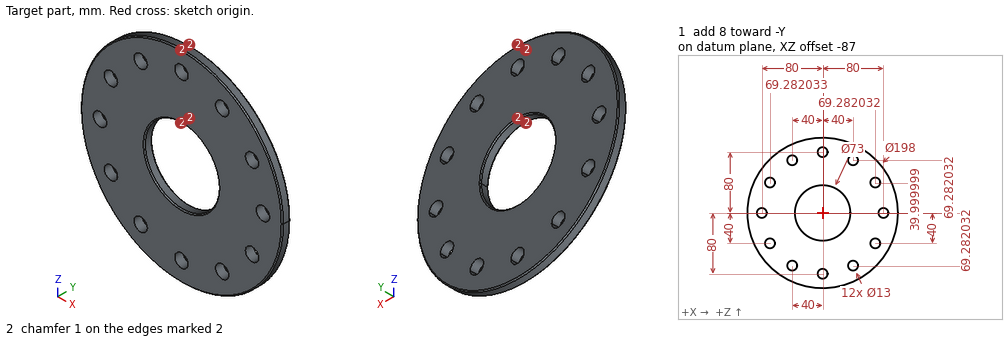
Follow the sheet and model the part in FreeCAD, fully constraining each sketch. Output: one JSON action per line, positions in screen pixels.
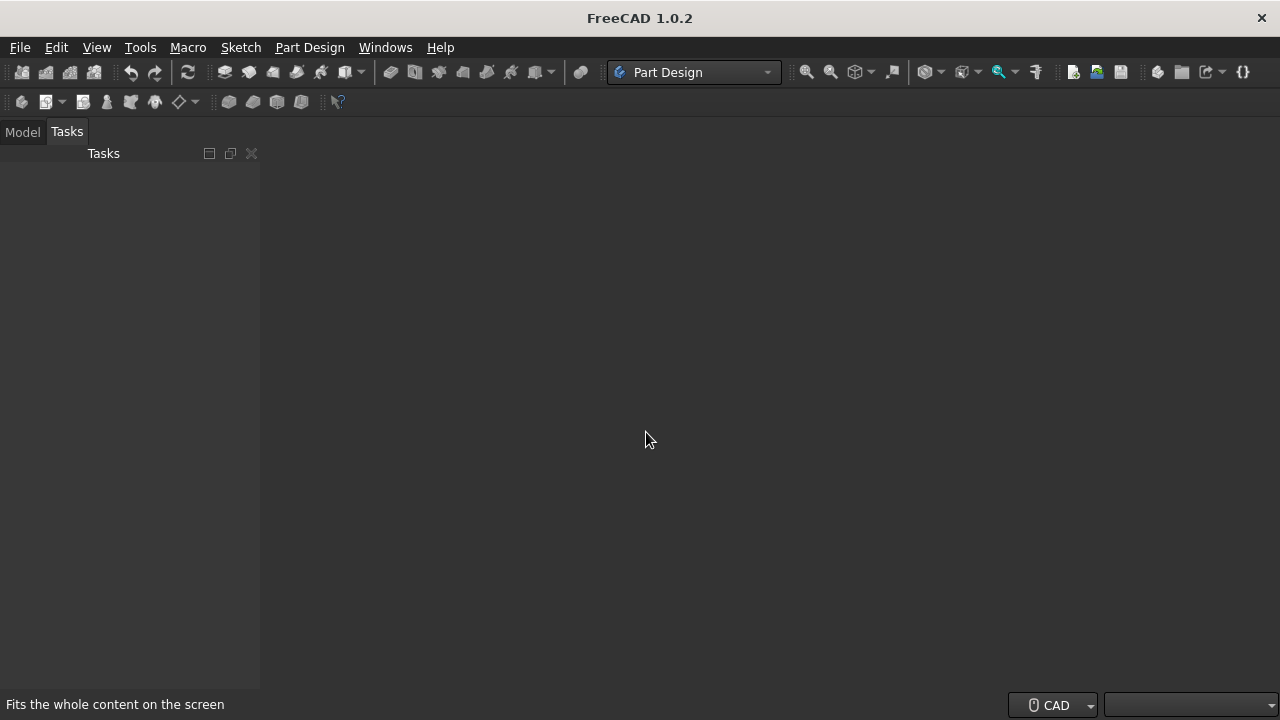
{"action": "key", "text": "ctrl+n"}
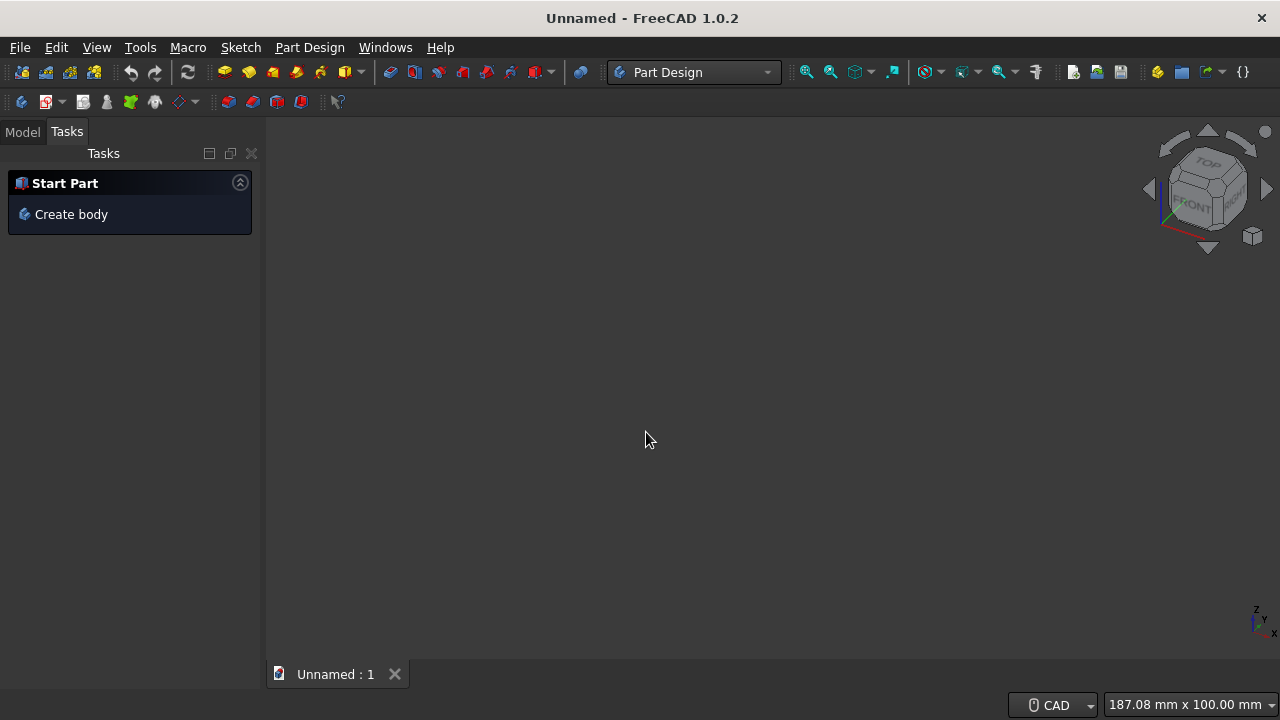
{"action": "left_click", "coordinate": [22, 102]}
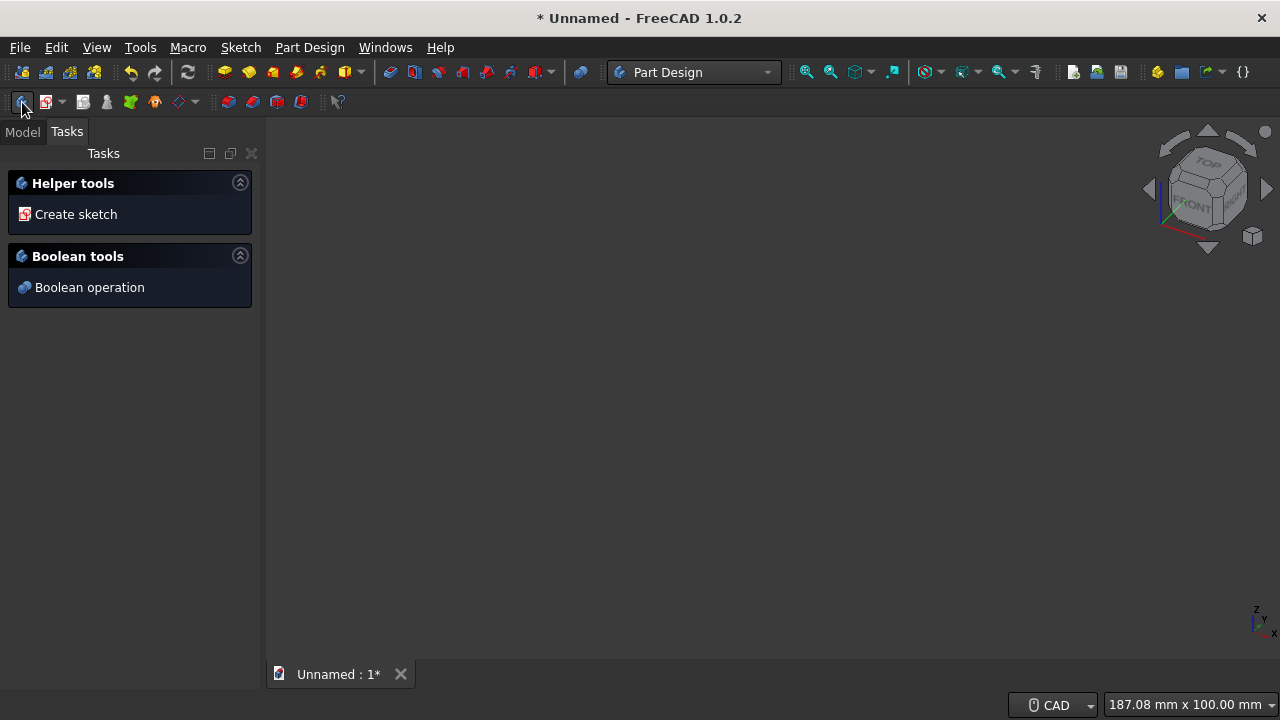
{"action": "left_click", "coordinate": [23, 131]}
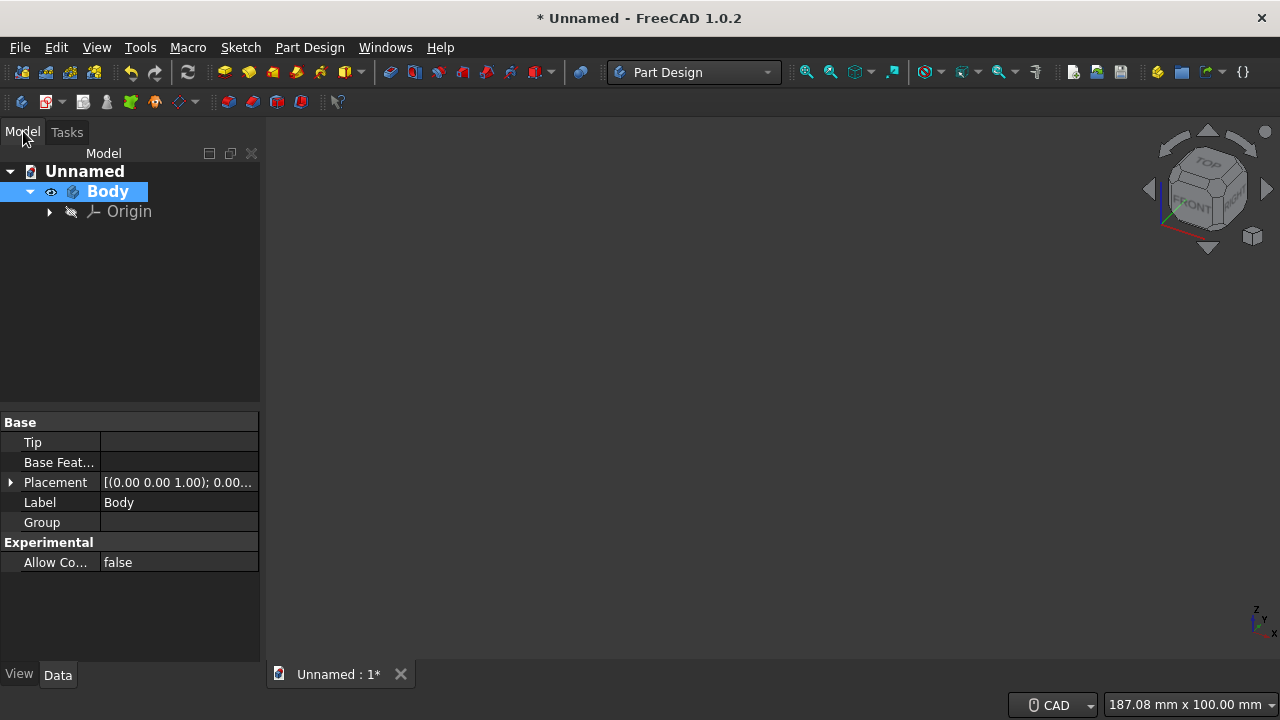
{"action": "left_click", "coordinate": [50, 212]}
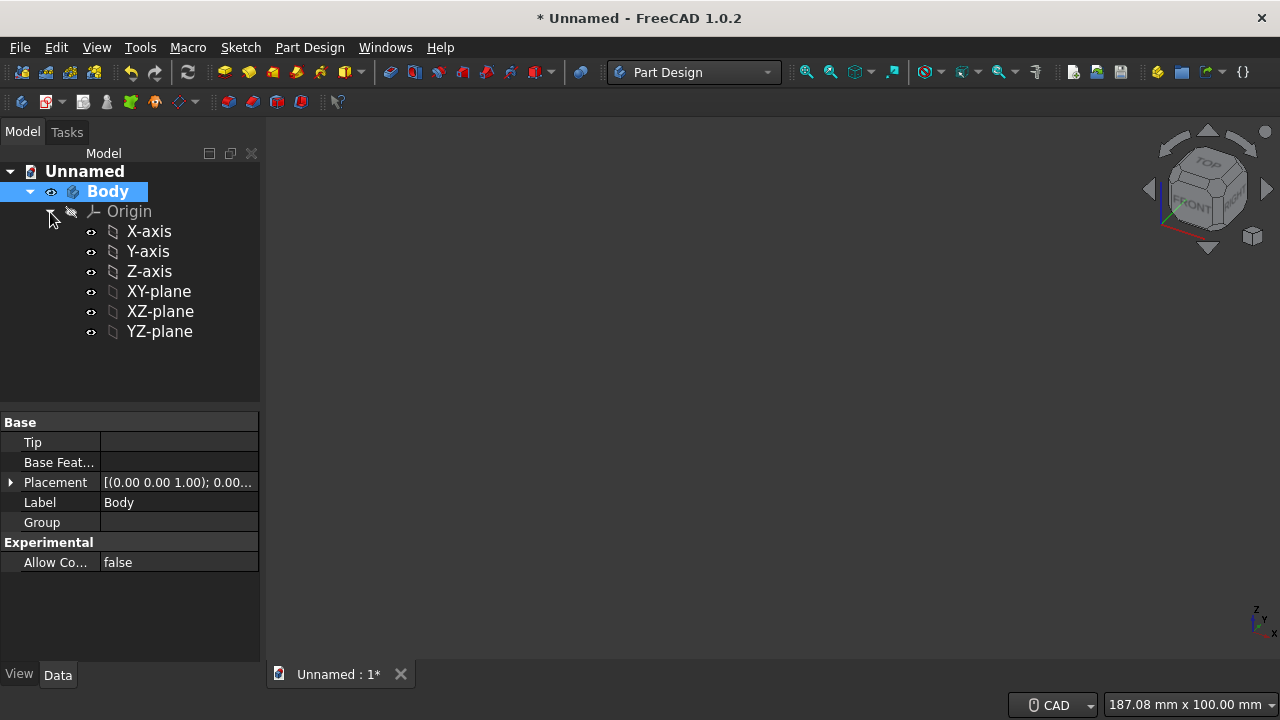
{"action": "left_click", "coordinate": [136, 312]}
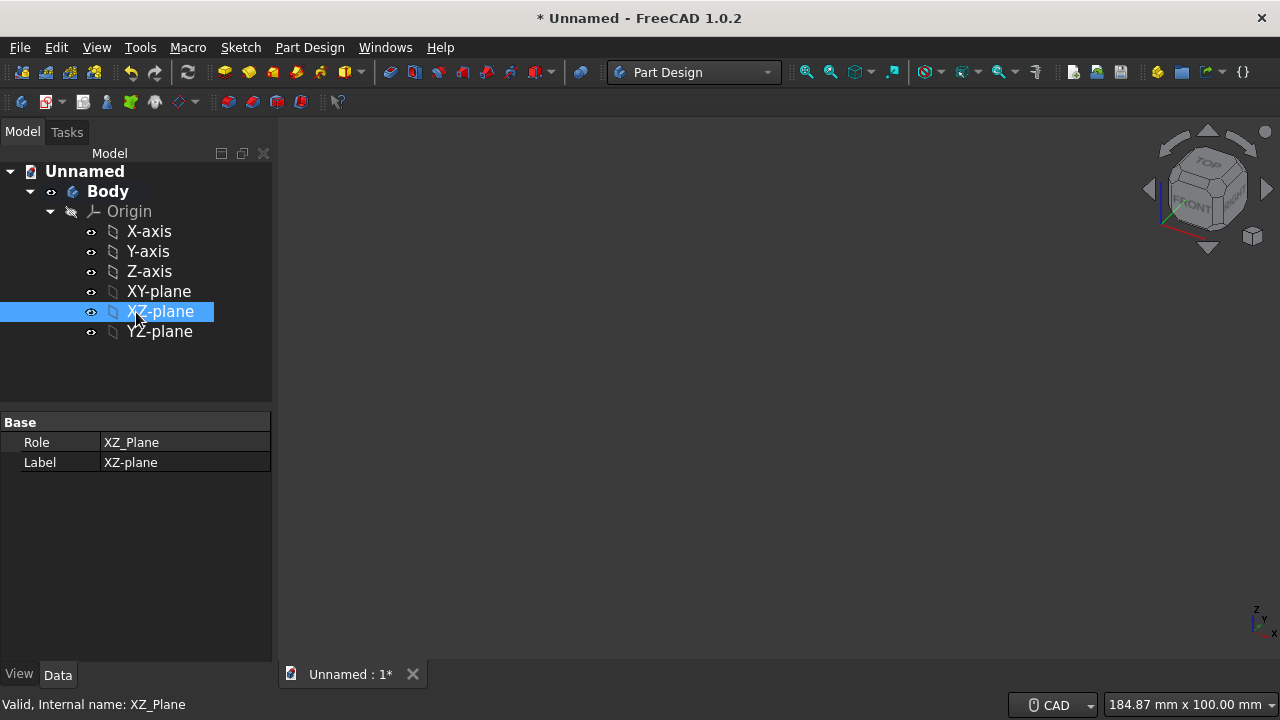
{"action": "left_click", "coordinate": [180, 102]}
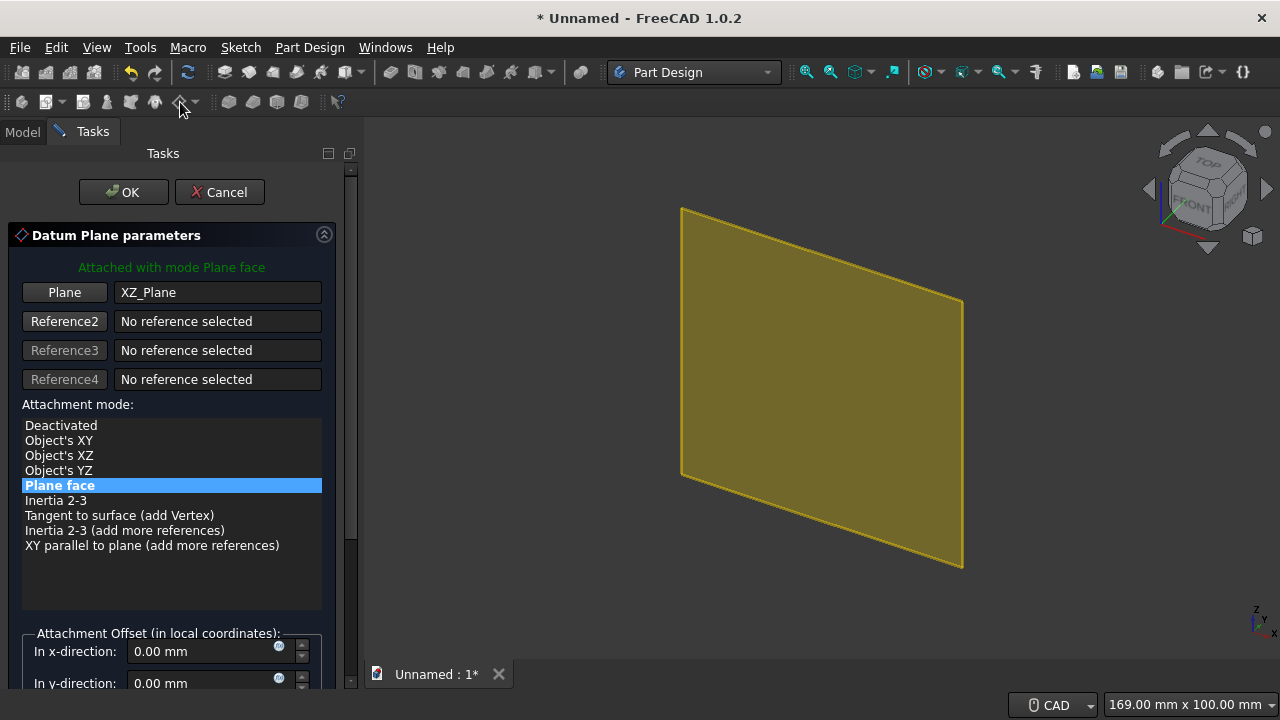
{"action": "scroll", "coordinate": [351, 426], "scroll_direction": "down", "scroll_amount": 2}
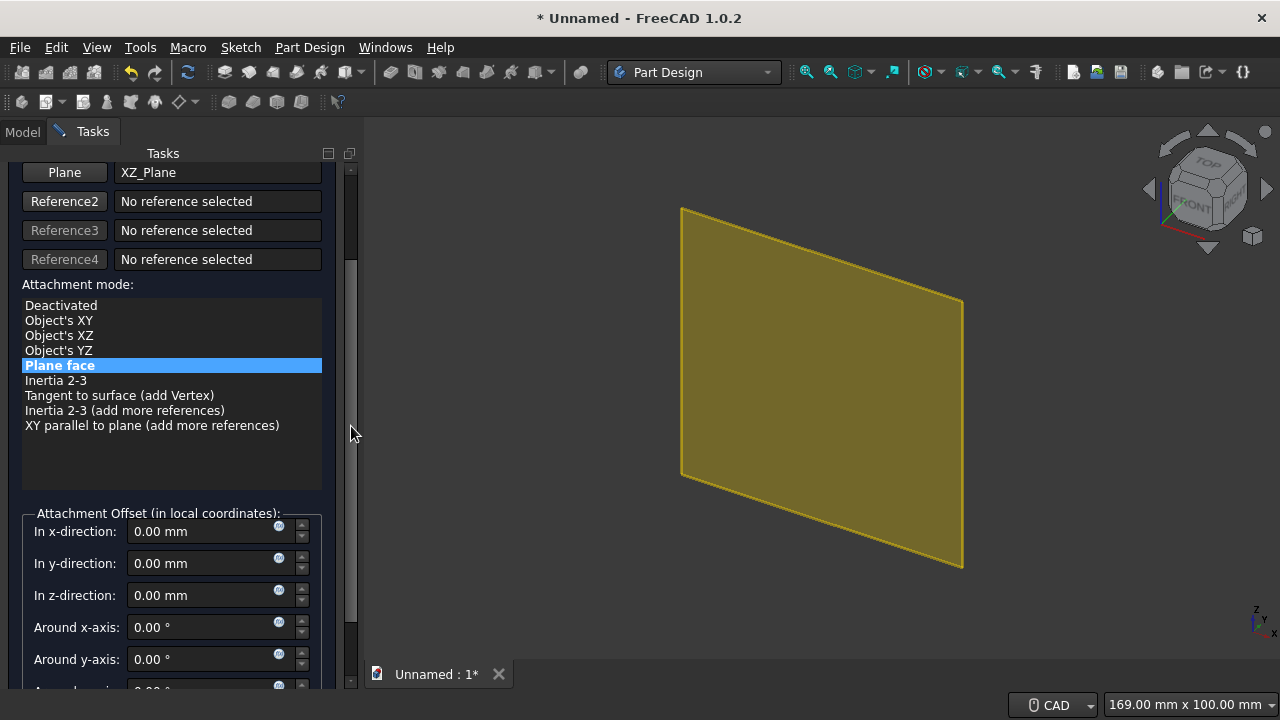
{"action": "triple_click", "coordinate": [210, 595]}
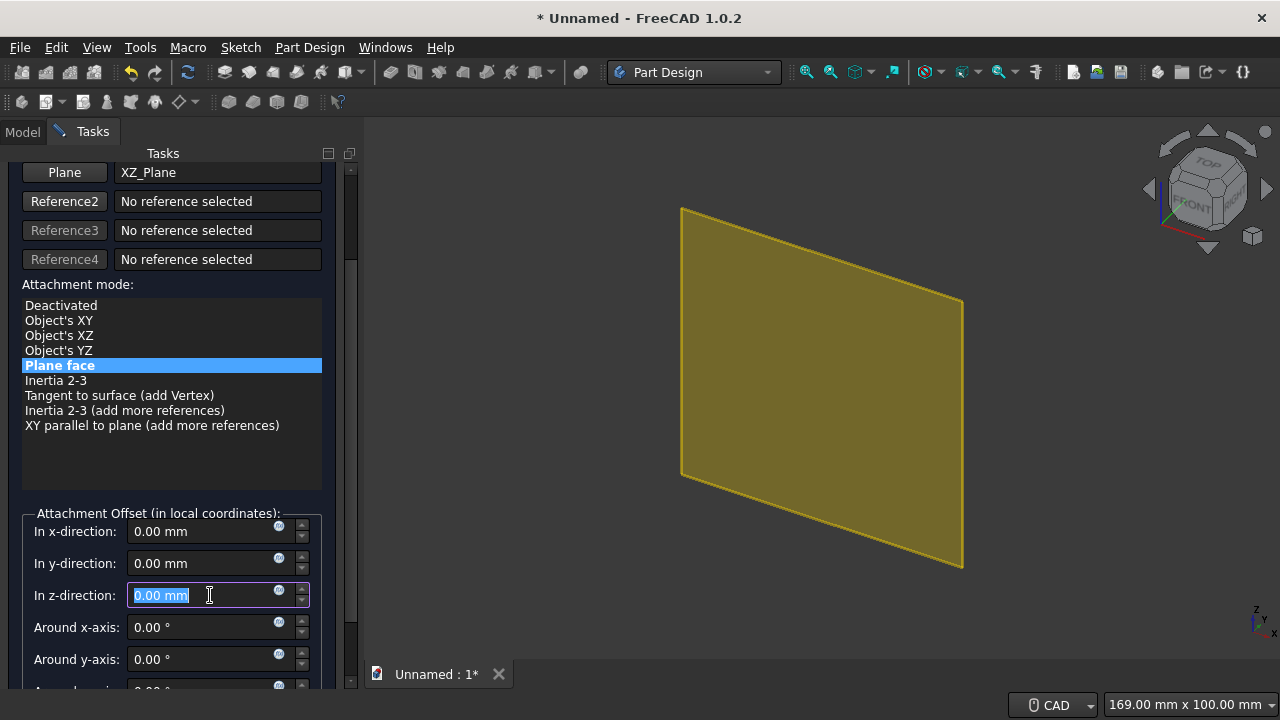
{"action": "type", "text": "-87"}
{"action": "key", "text": "Tab"}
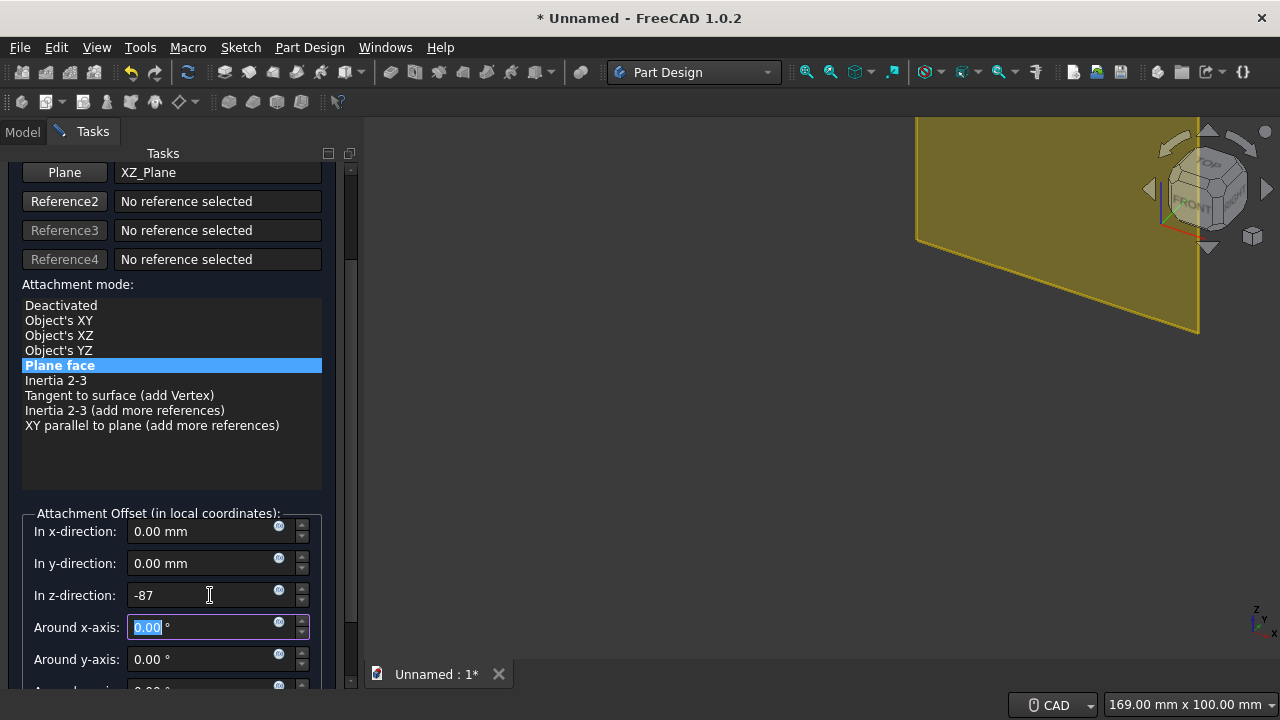
{"action": "scroll", "coordinate": [351, 426], "scroll_direction": "up", "scroll_amount": 3}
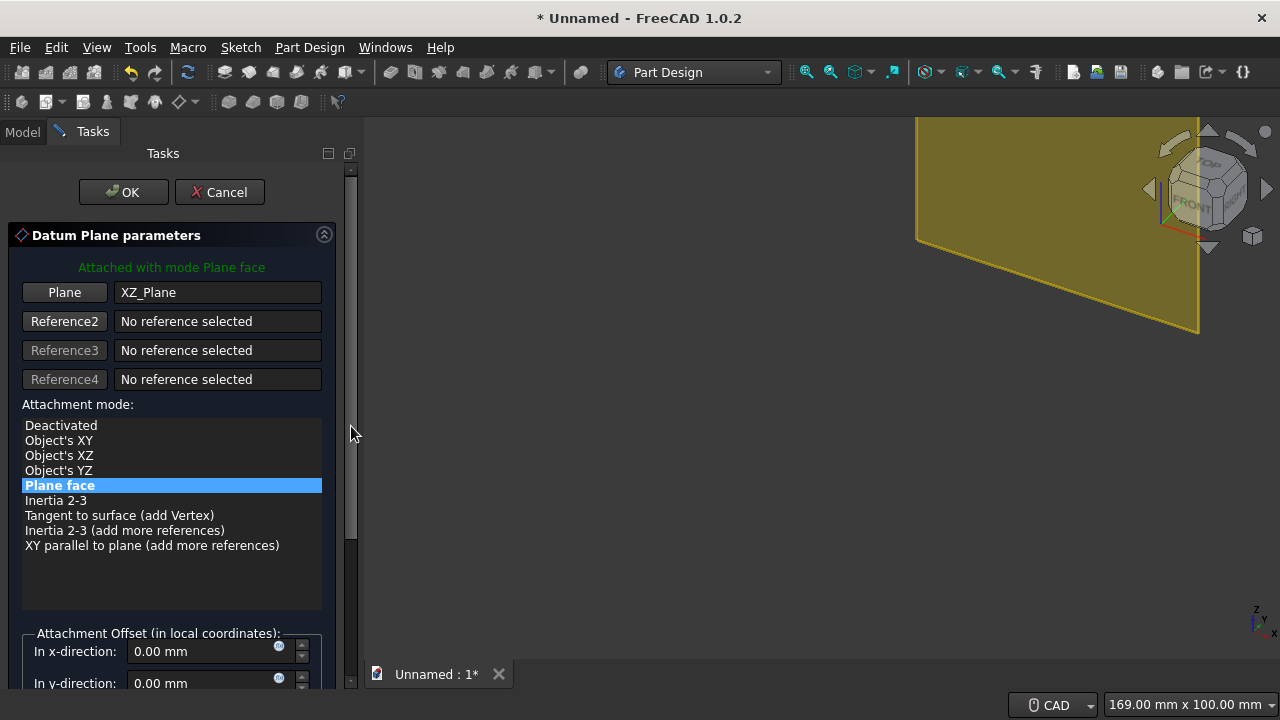
{"action": "left_click", "coordinate": [124, 192]}